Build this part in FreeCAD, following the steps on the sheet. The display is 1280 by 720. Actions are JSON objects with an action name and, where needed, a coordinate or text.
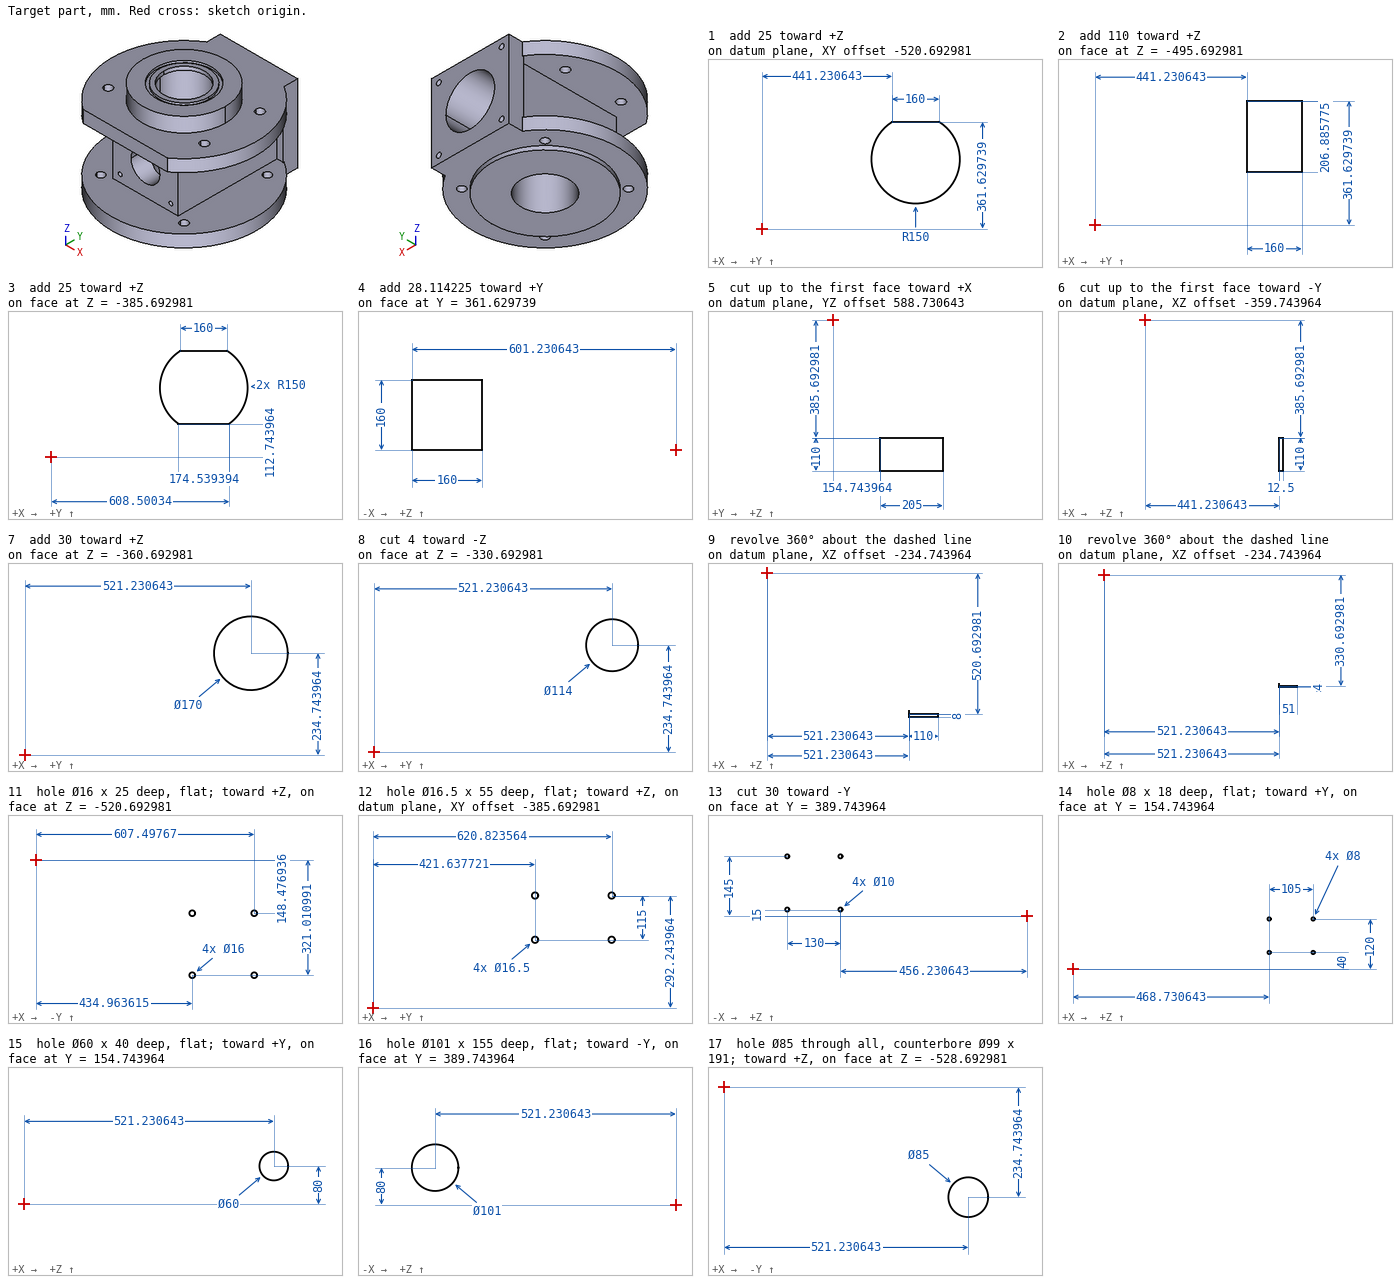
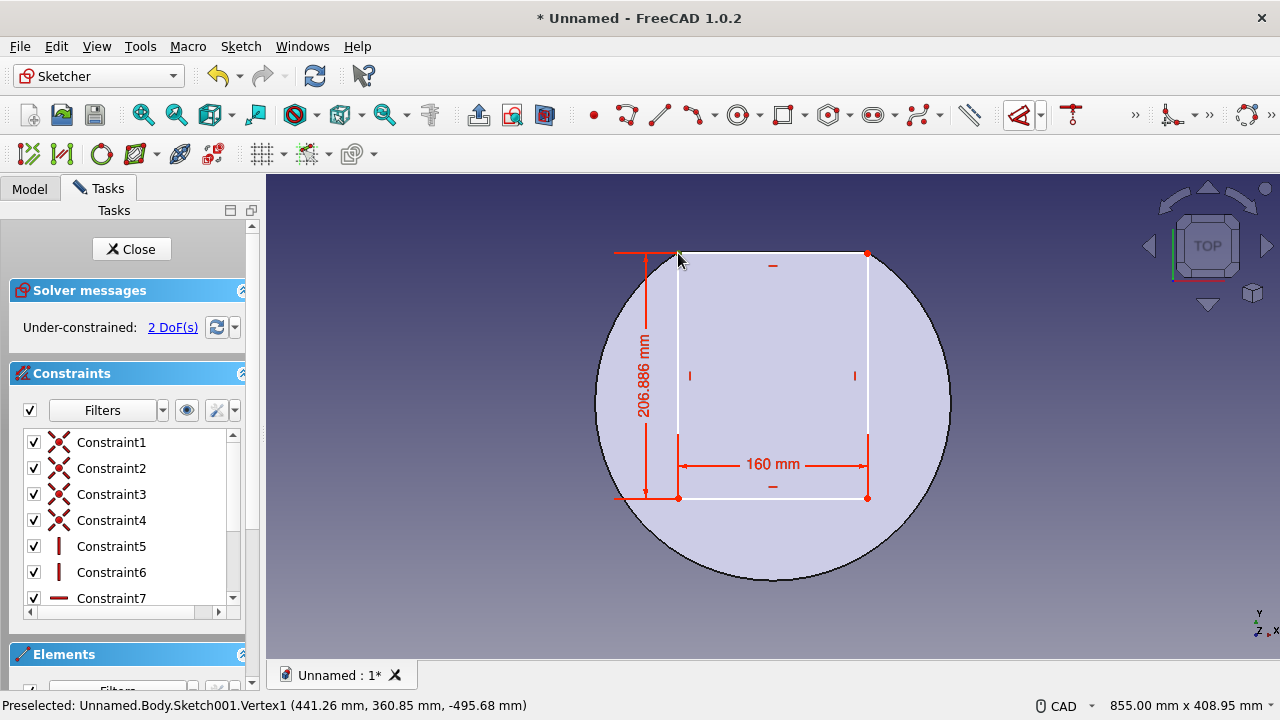
{"action": "left_click", "coordinate": [1040, 116]}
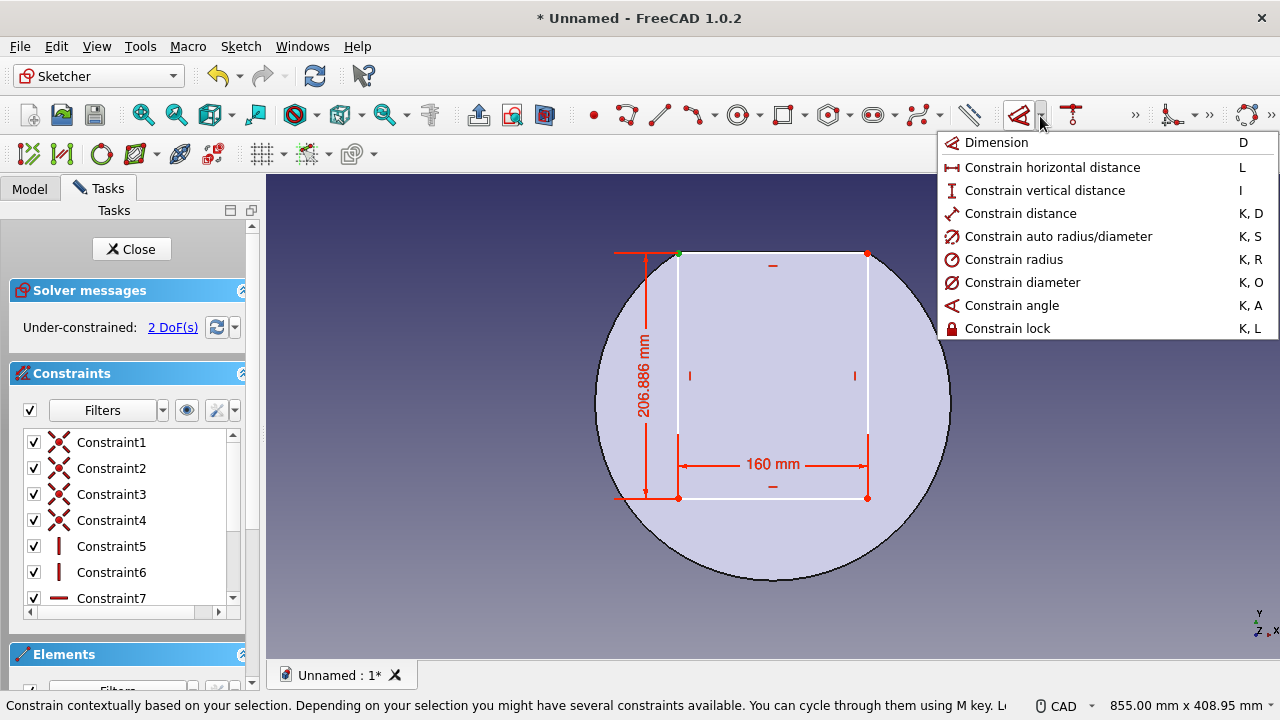
{"action": "left_click", "coordinate": [1108, 168]}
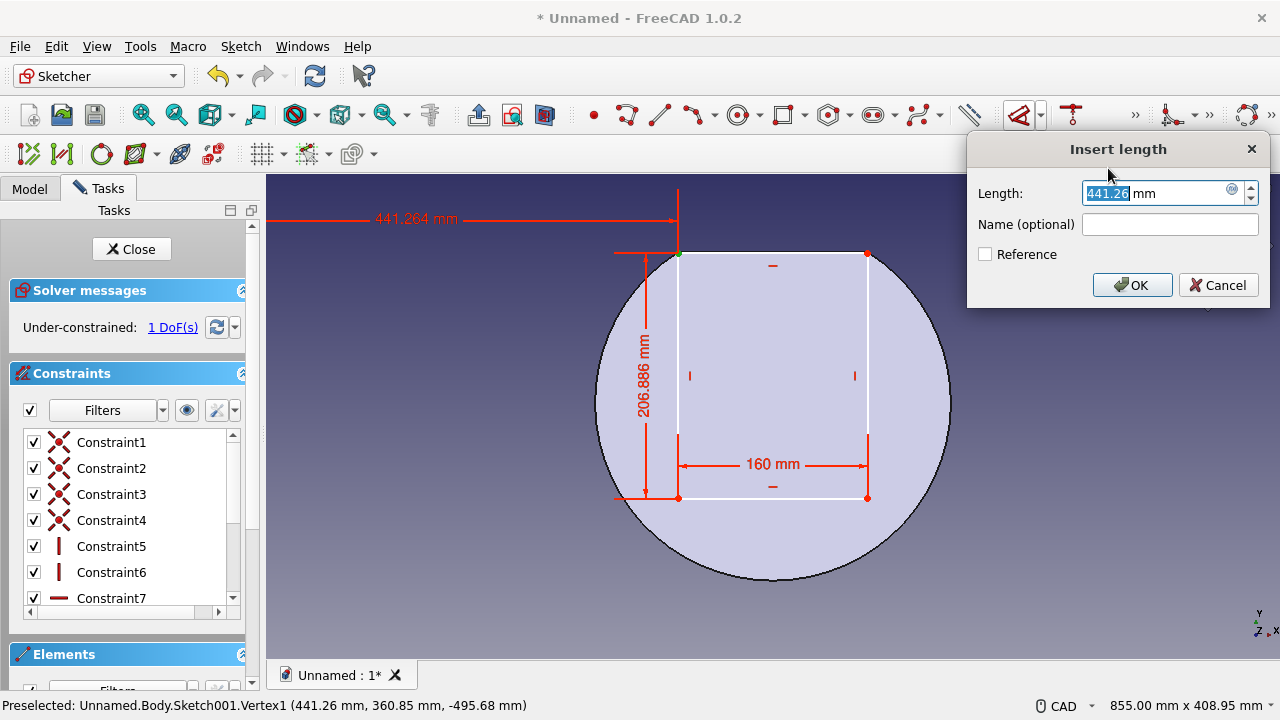
{"action": "type", "text": "441.230643"}
{"action": "key", "text": "Return"}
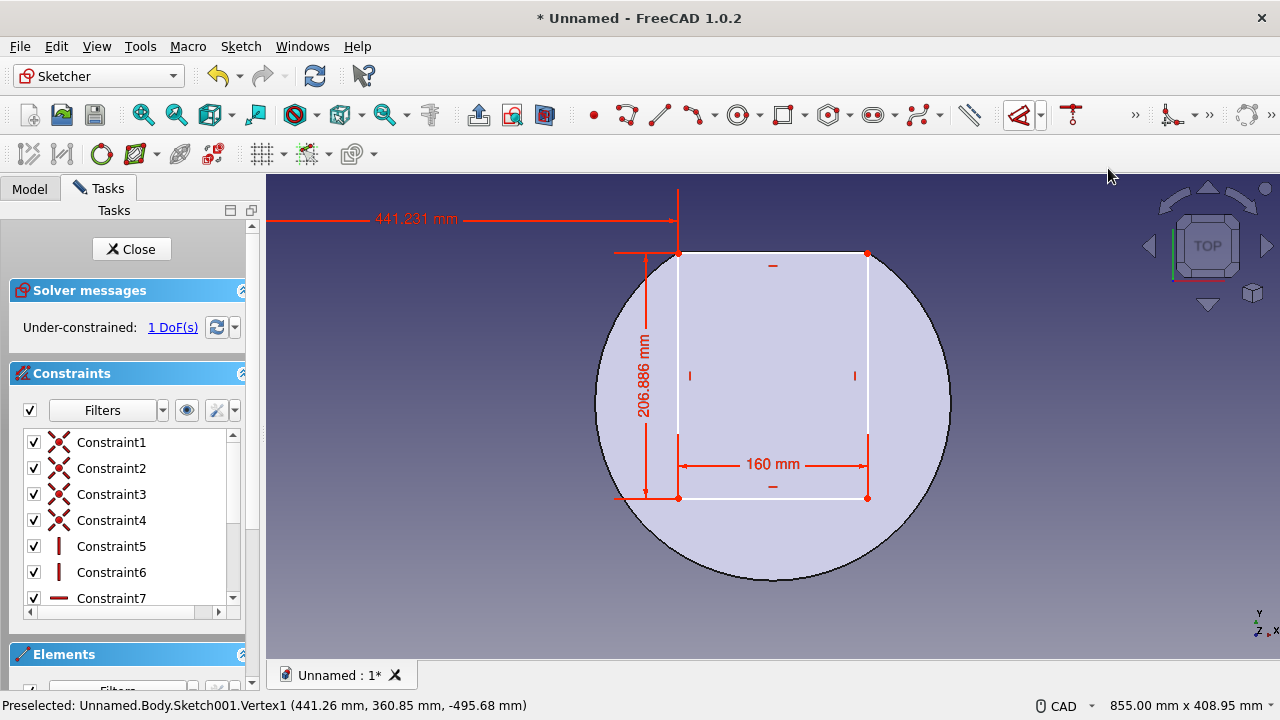
{"action": "left_click", "coordinate": [678, 253]}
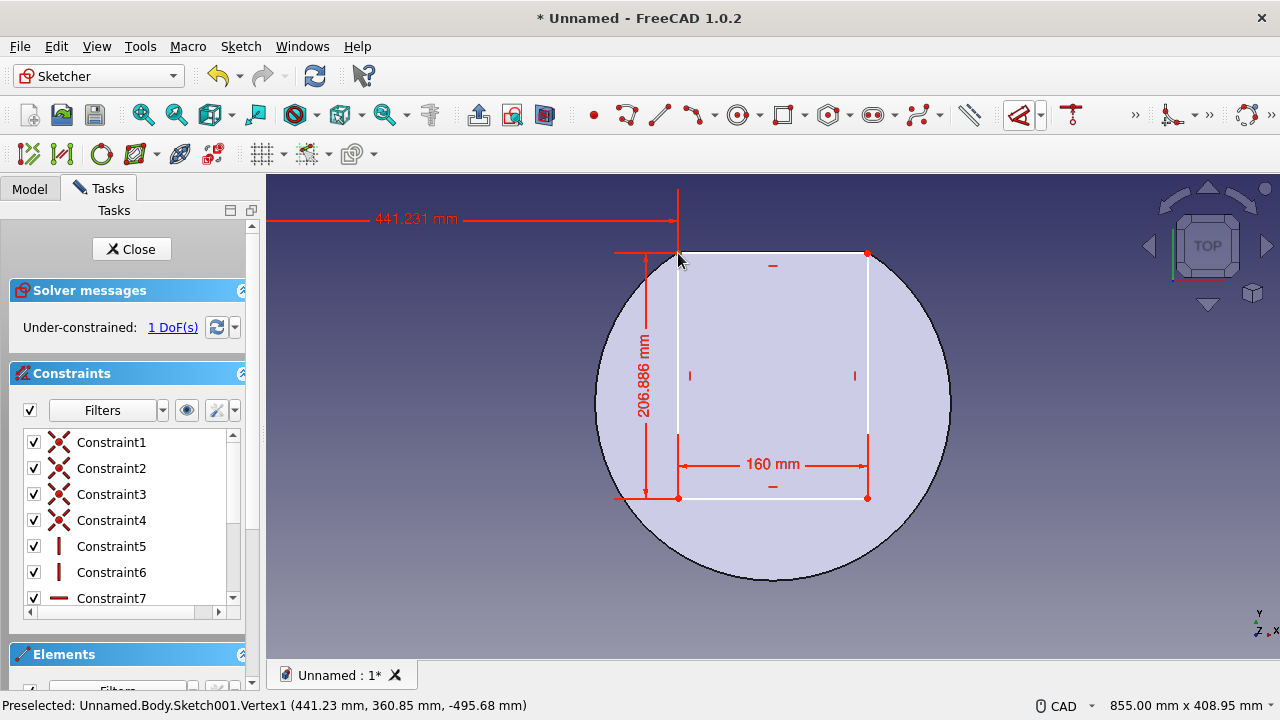
{"action": "left_click", "coordinate": [1040, 116]}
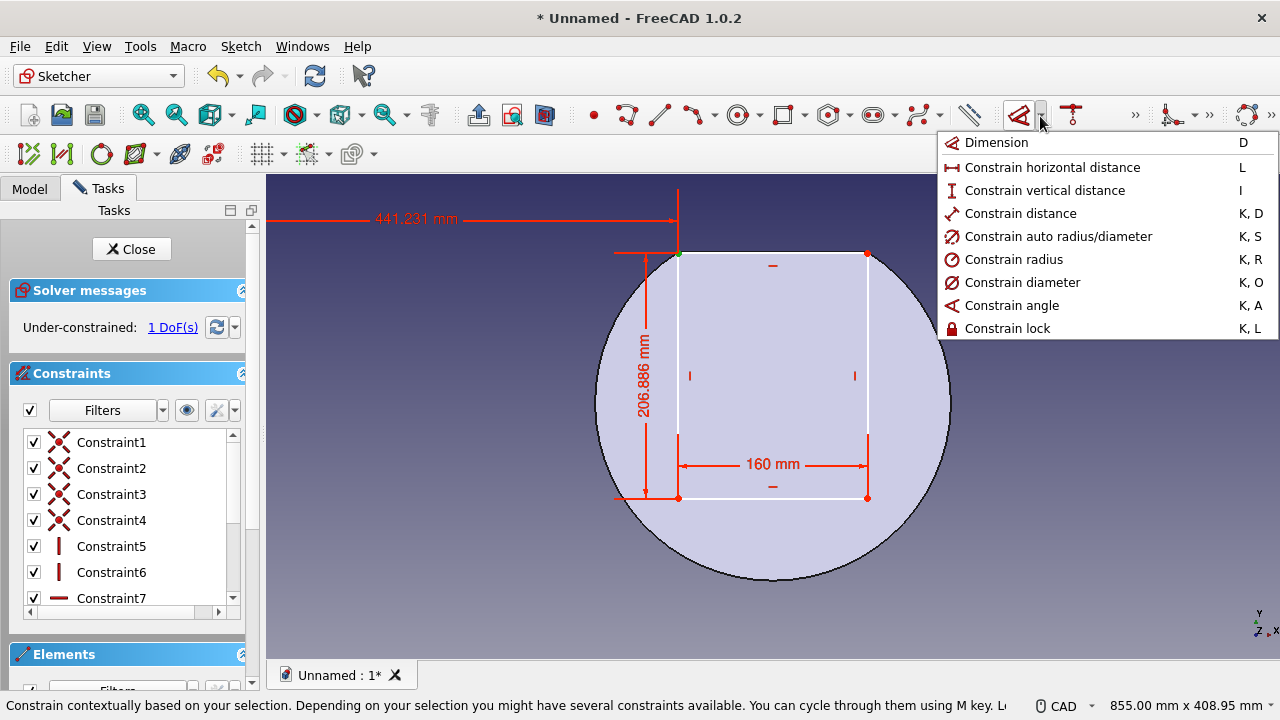
{"action": "left_click", "coordinate": [1108, 190]}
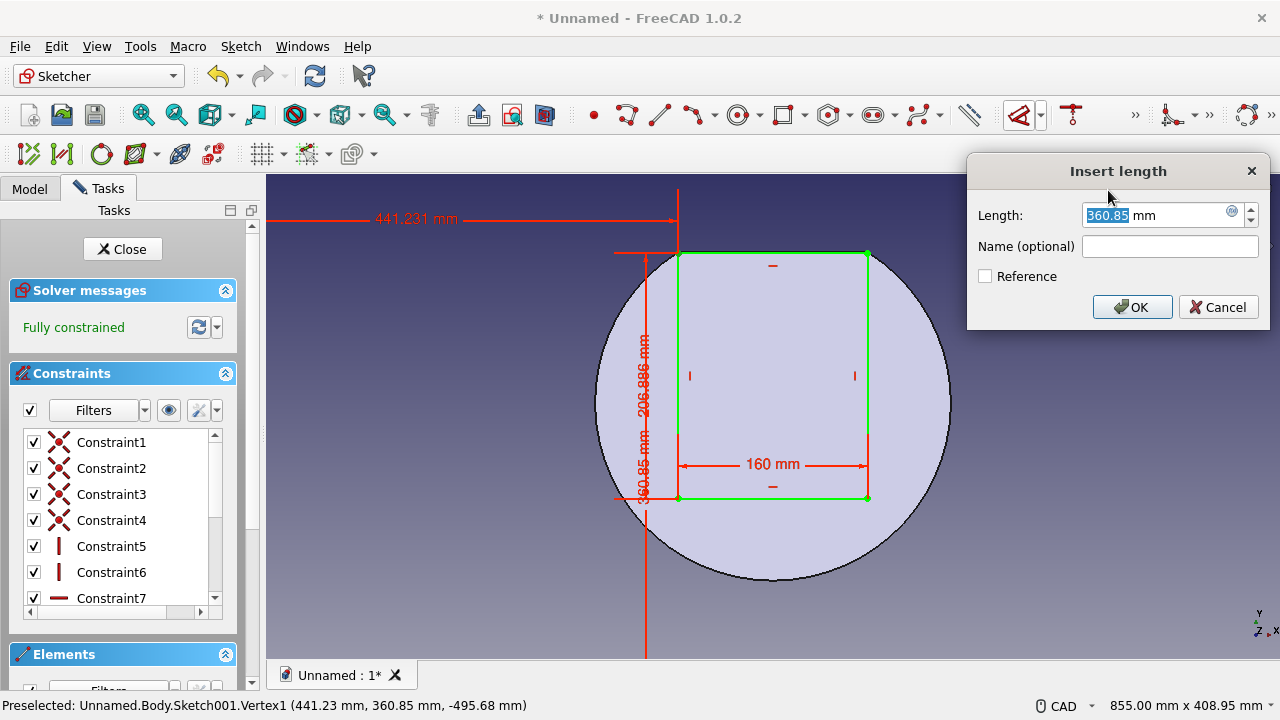
{"action": "type", "text": "361.629739"}
{"action": "key", "text": "Return"}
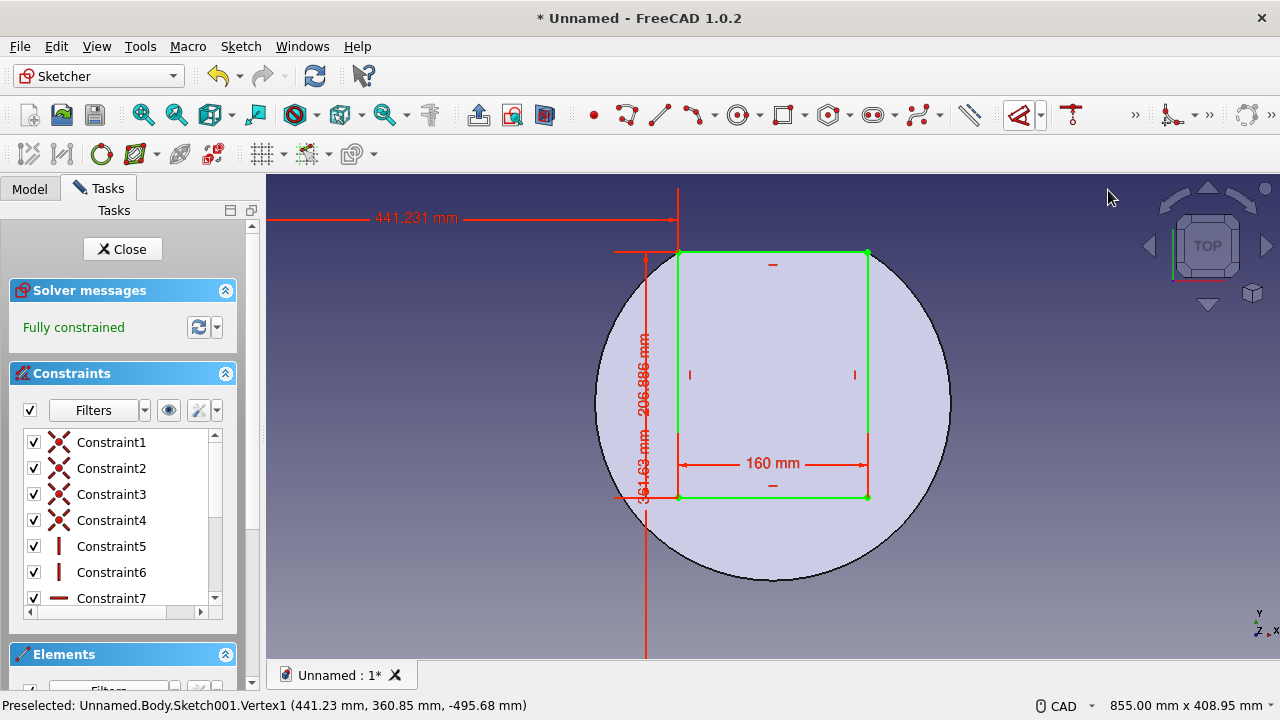
{"action": "left_click", "coordinate": [123, 249]}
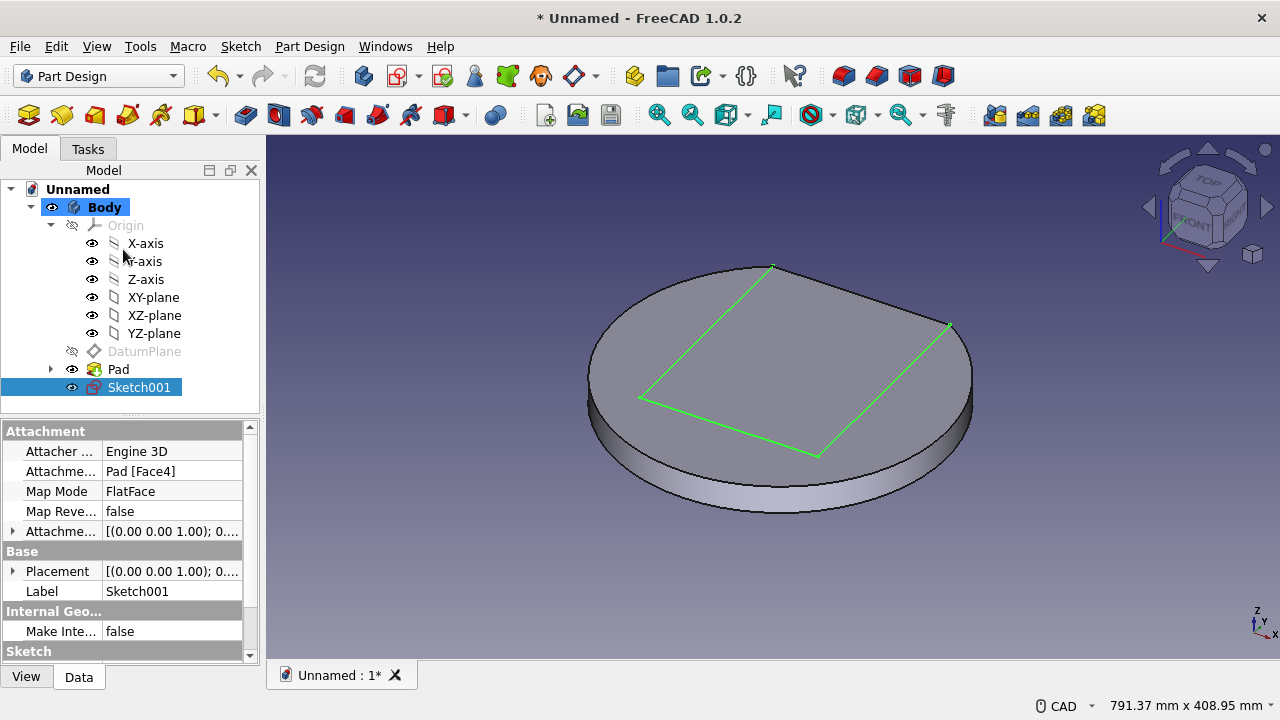
{"action": "left_click", "coordinate": [29, 116]}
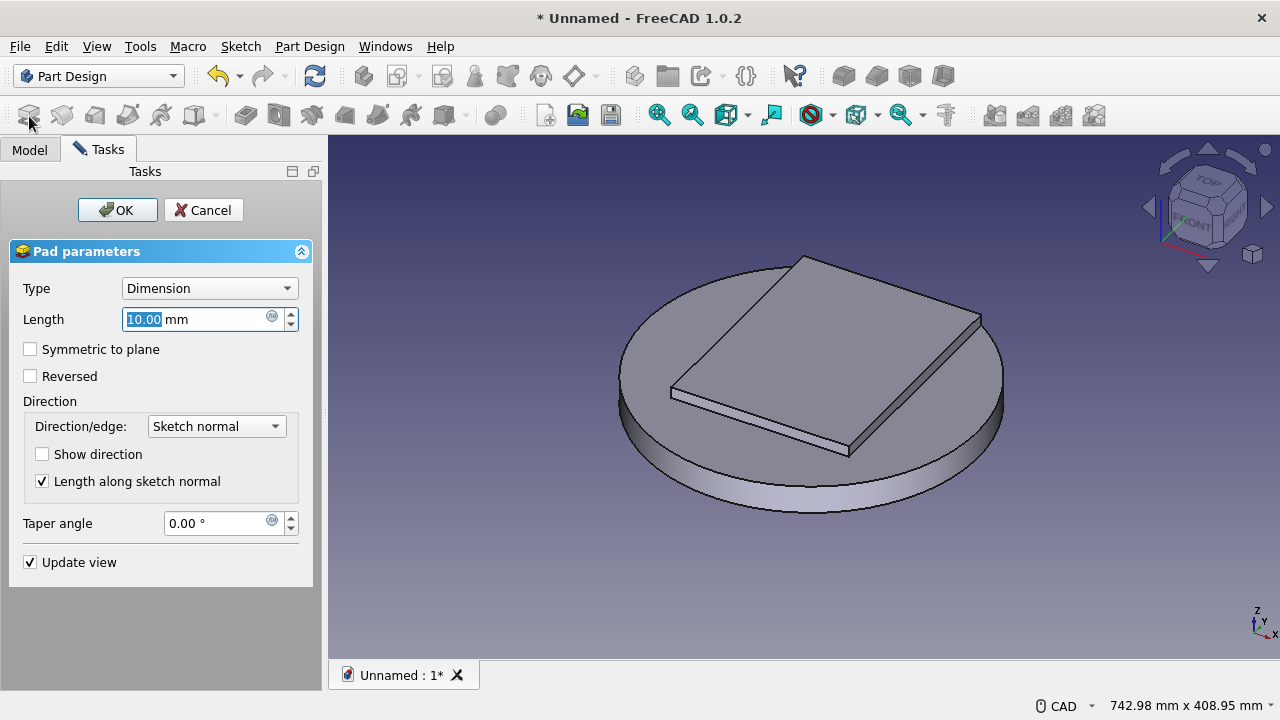
{"action": "type", "text": "110"}
{"action": "key", "text": "Tab"}